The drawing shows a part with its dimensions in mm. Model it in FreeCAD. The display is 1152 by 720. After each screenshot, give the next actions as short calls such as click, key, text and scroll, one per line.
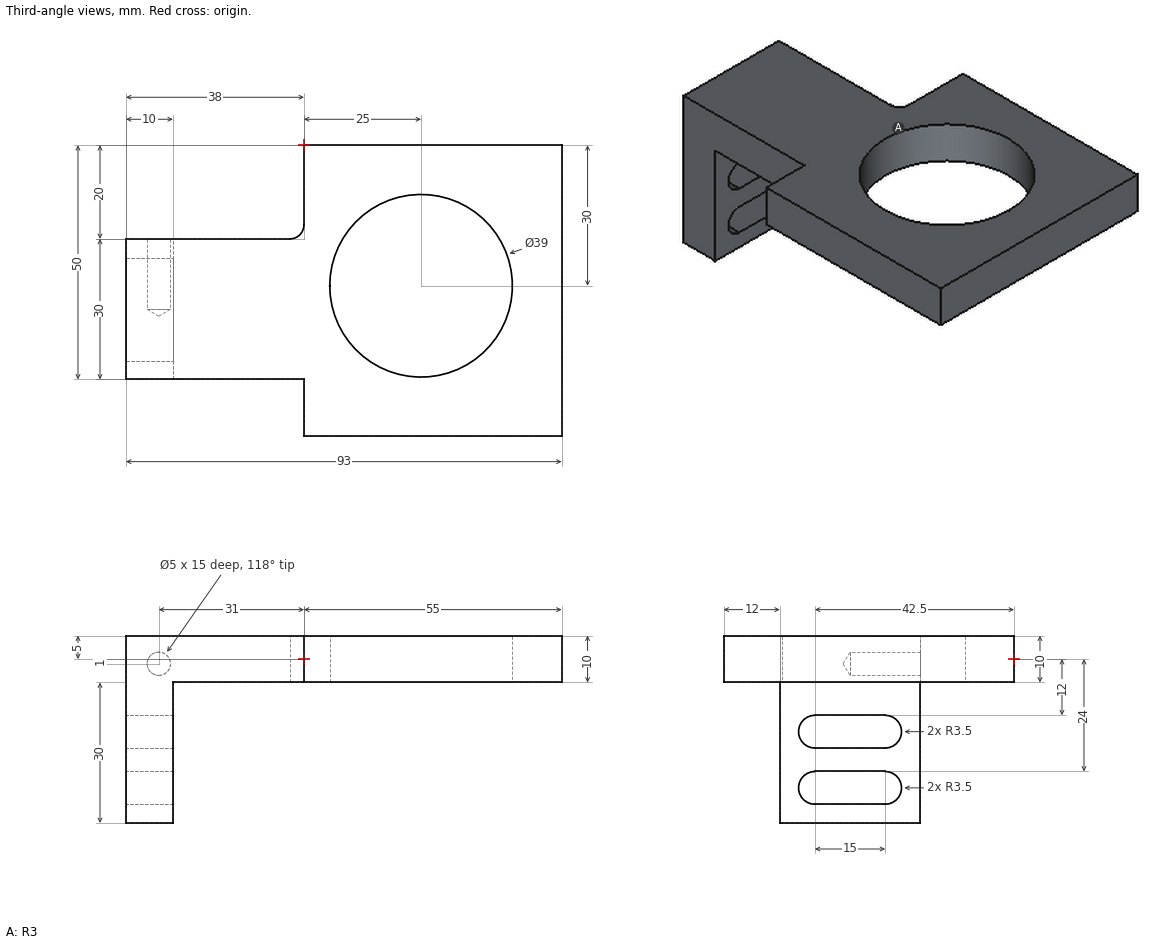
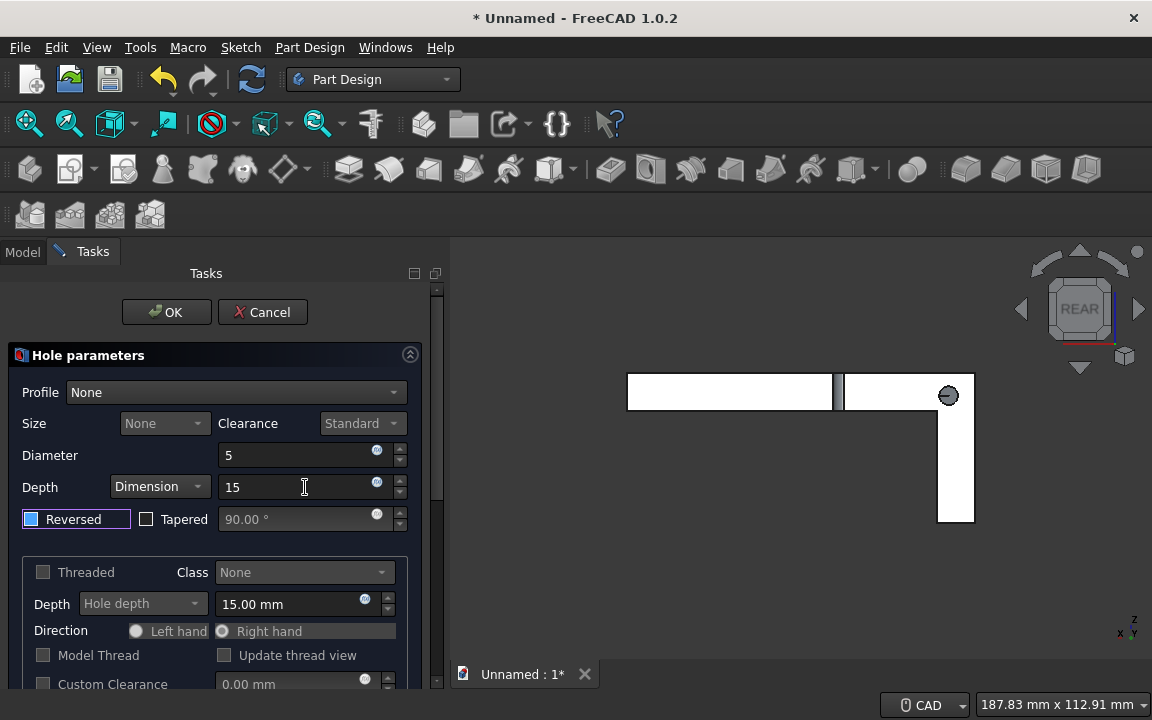
click(167, 312)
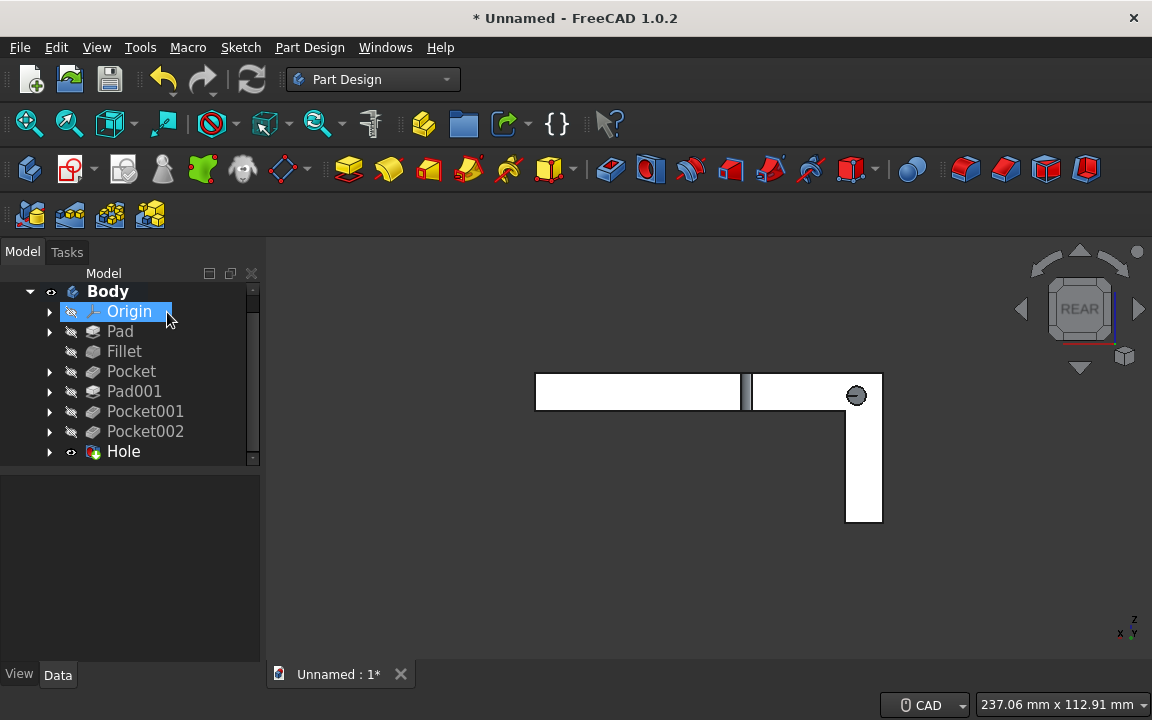
key(v)
key(f)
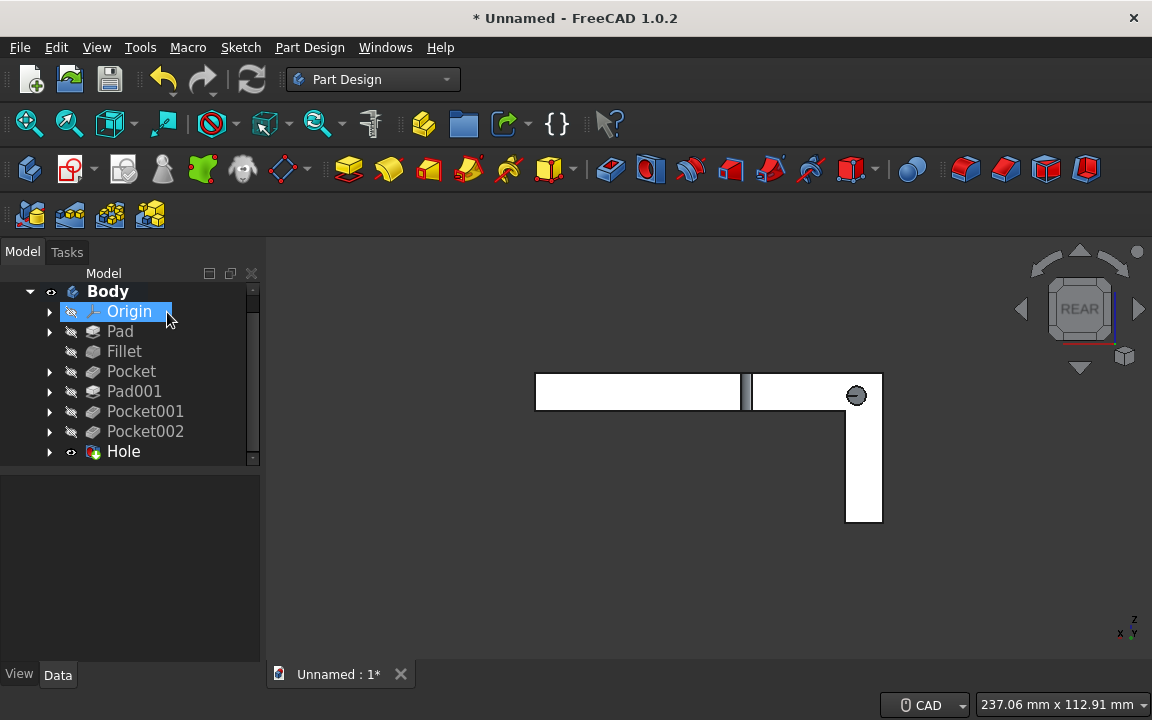
key(0)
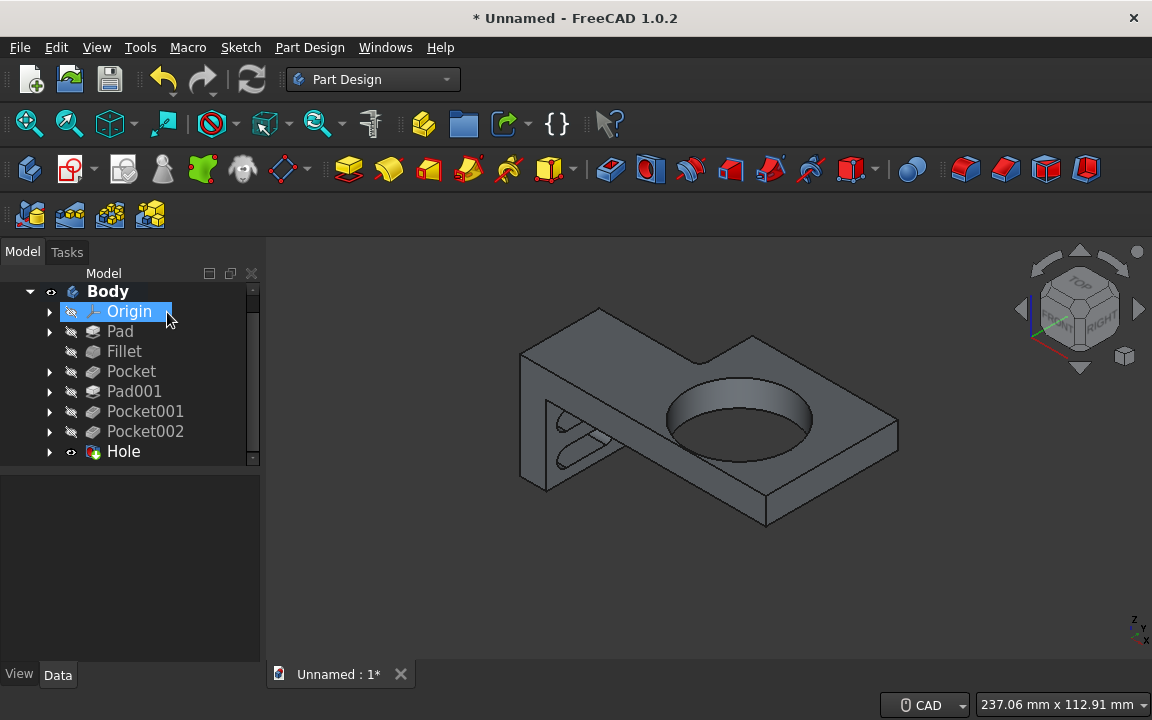
click(538, 389)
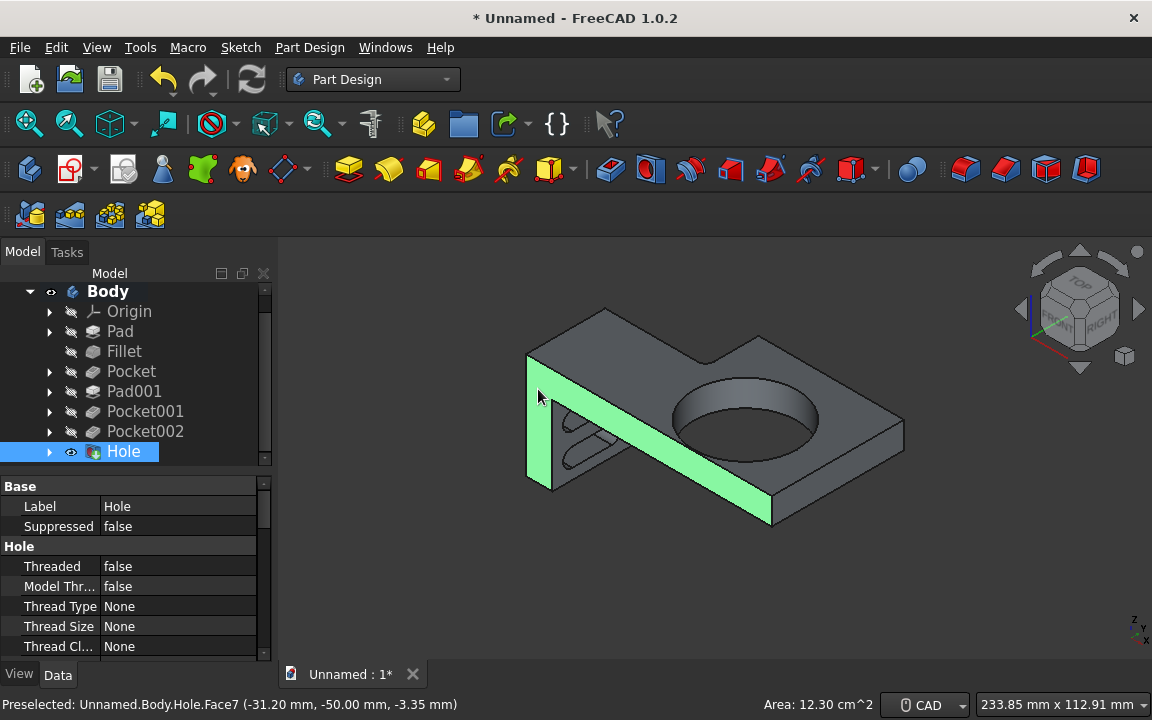
click(70, 170)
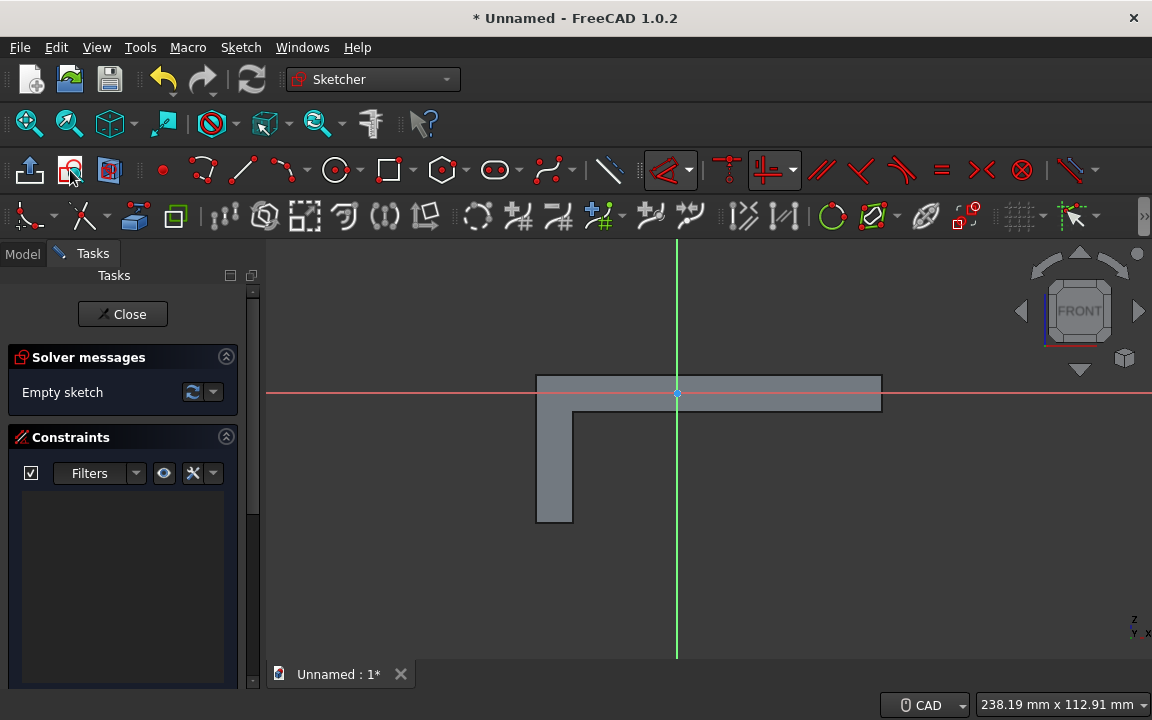
scroll(893, 348, up, 4)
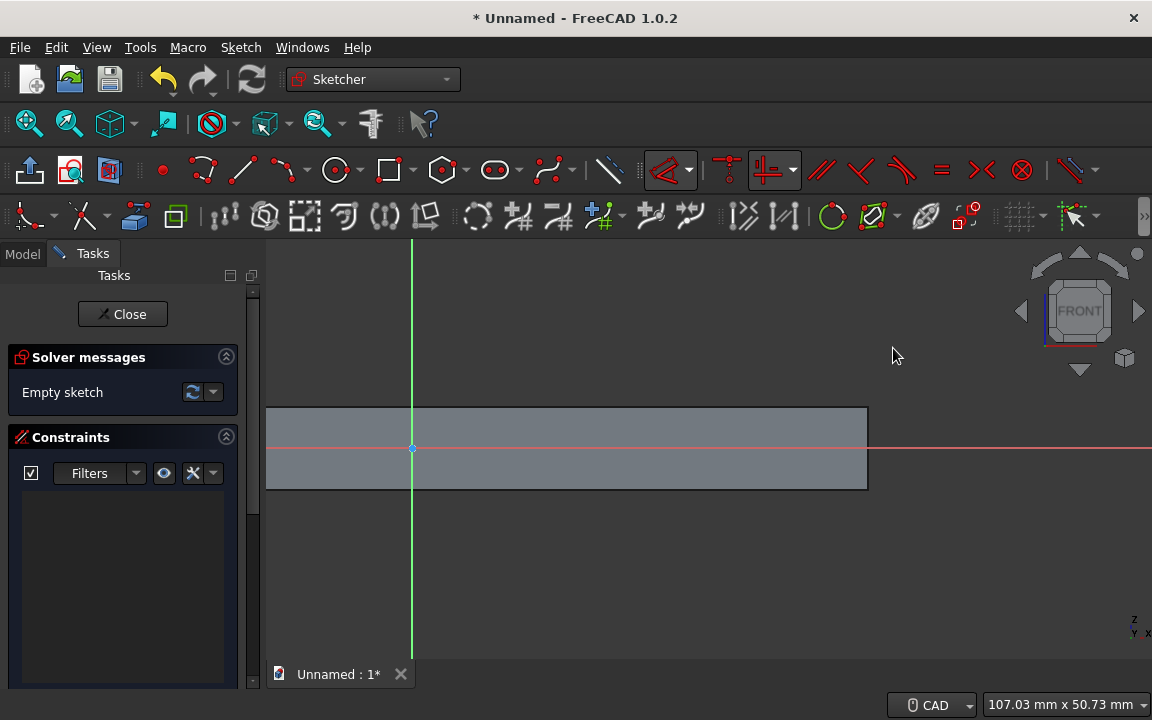
click(390, 170)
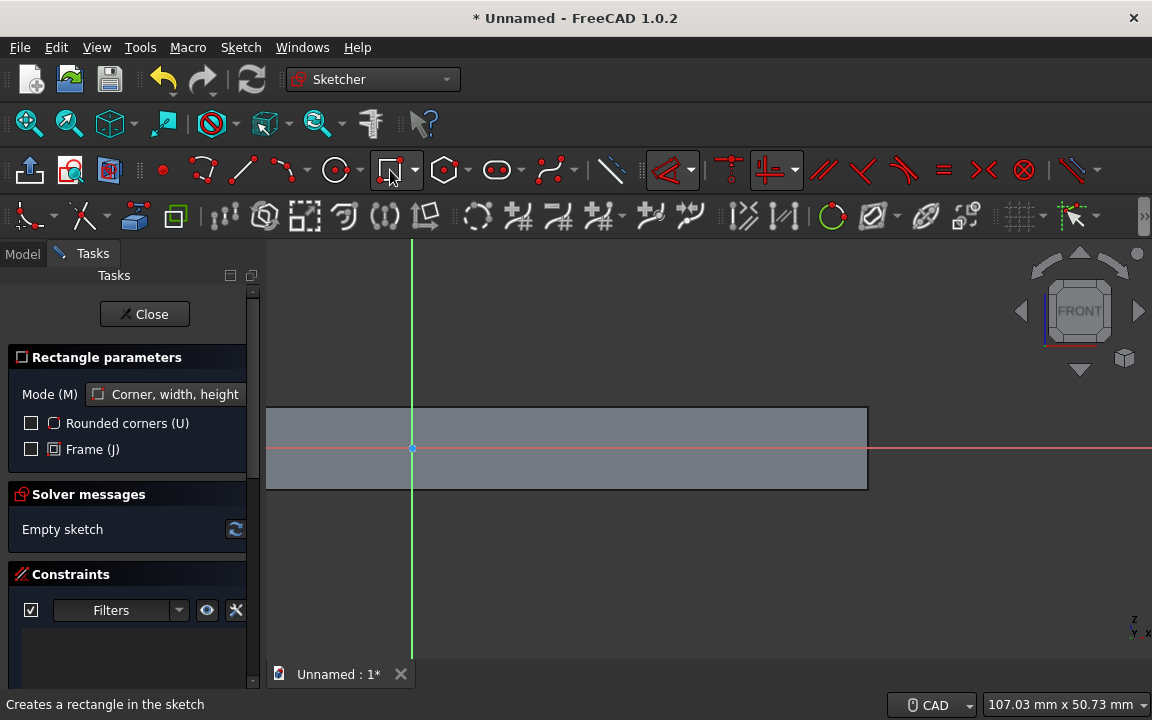
click(412, 407)
move(868, 490)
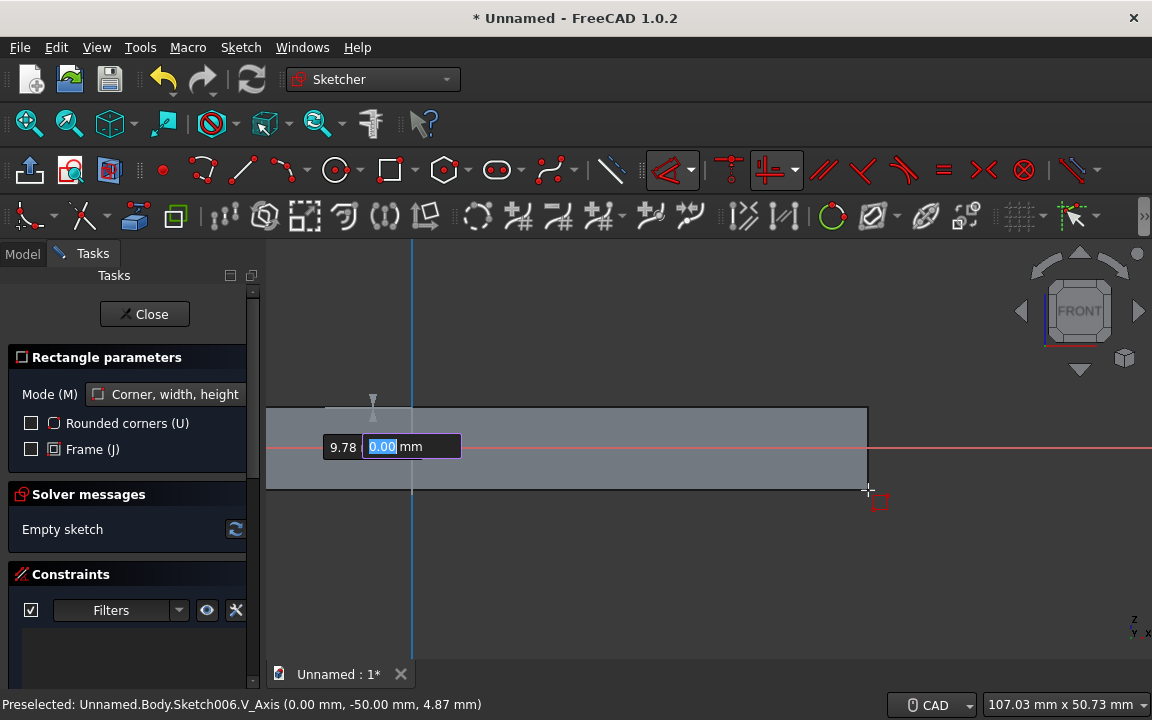
text(55)
key(Tab)
text(10)
key(Return)
key(Escape)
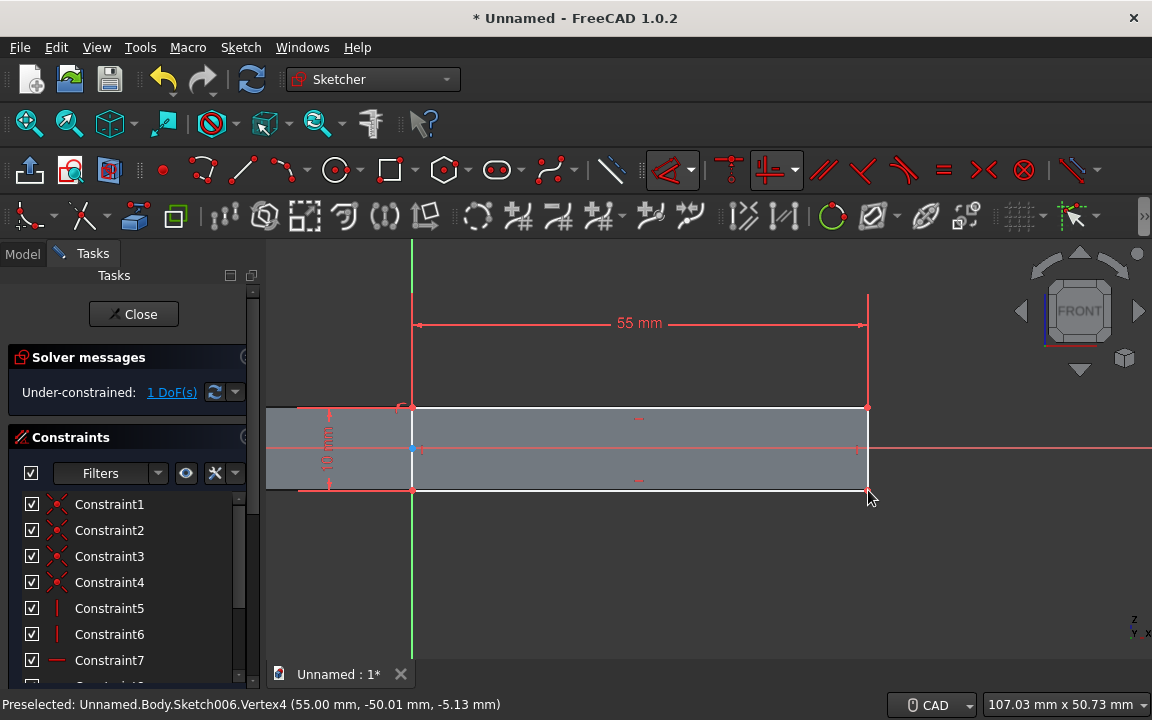
click(412, 408)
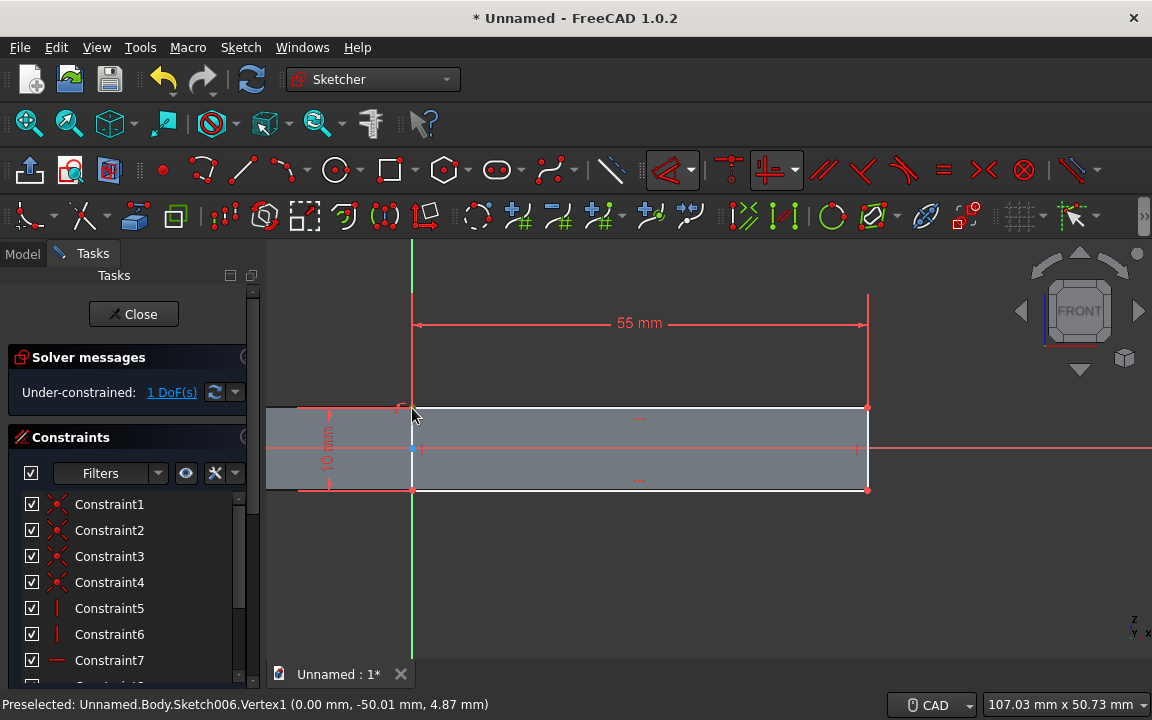
key(i)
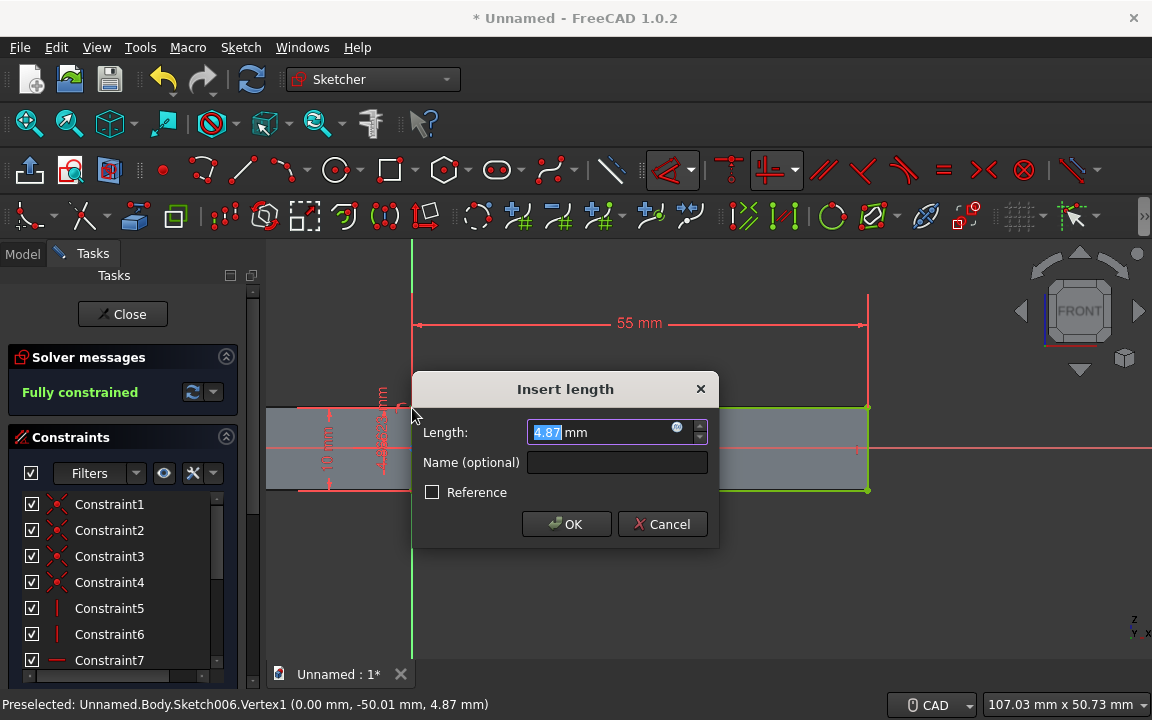
text(5)
key(Return)